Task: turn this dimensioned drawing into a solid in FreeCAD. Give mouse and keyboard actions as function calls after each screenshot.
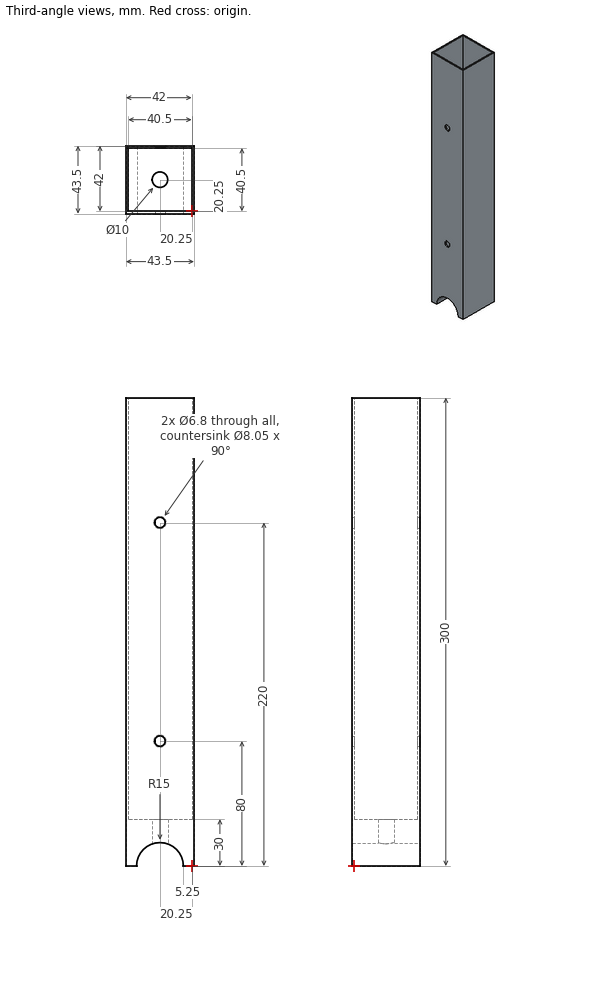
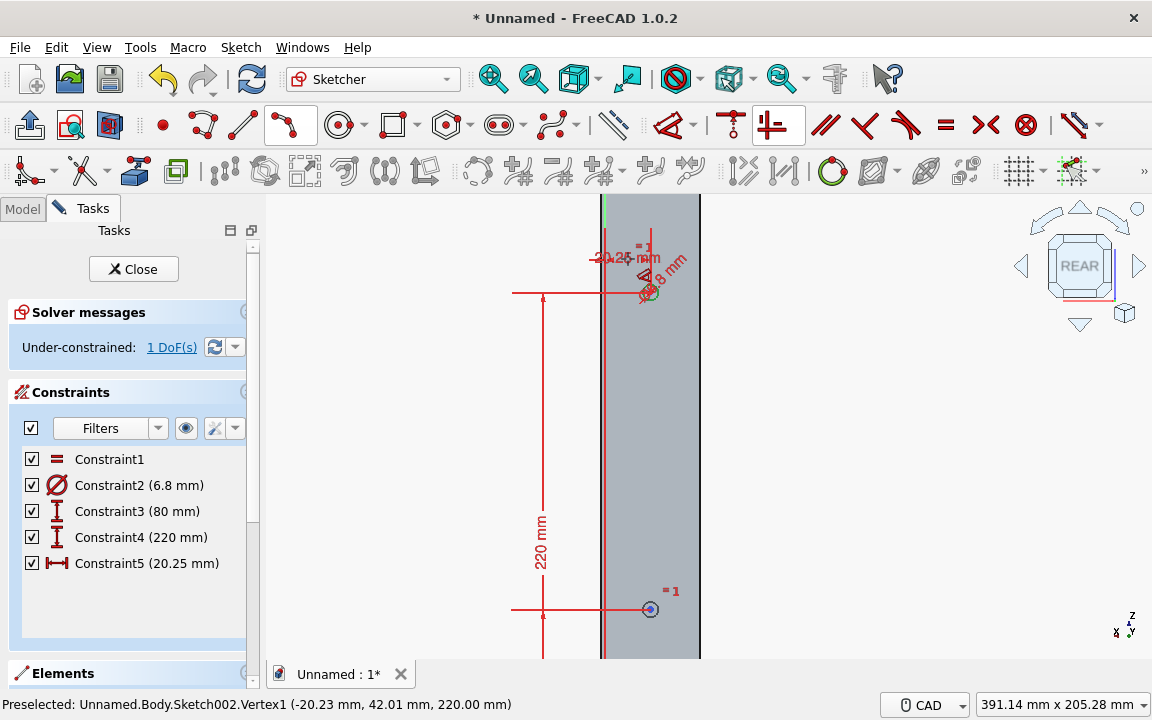
click(651, 610)
click(628, 576)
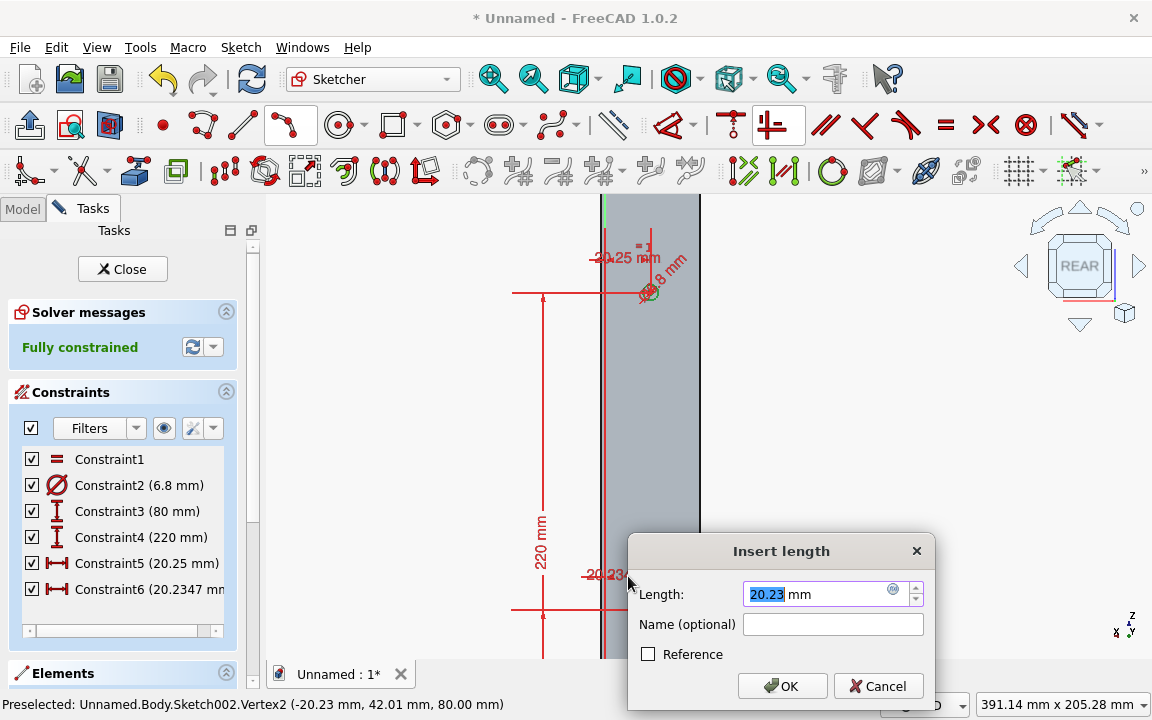
text(20.25)
key(Return)
key(Escape)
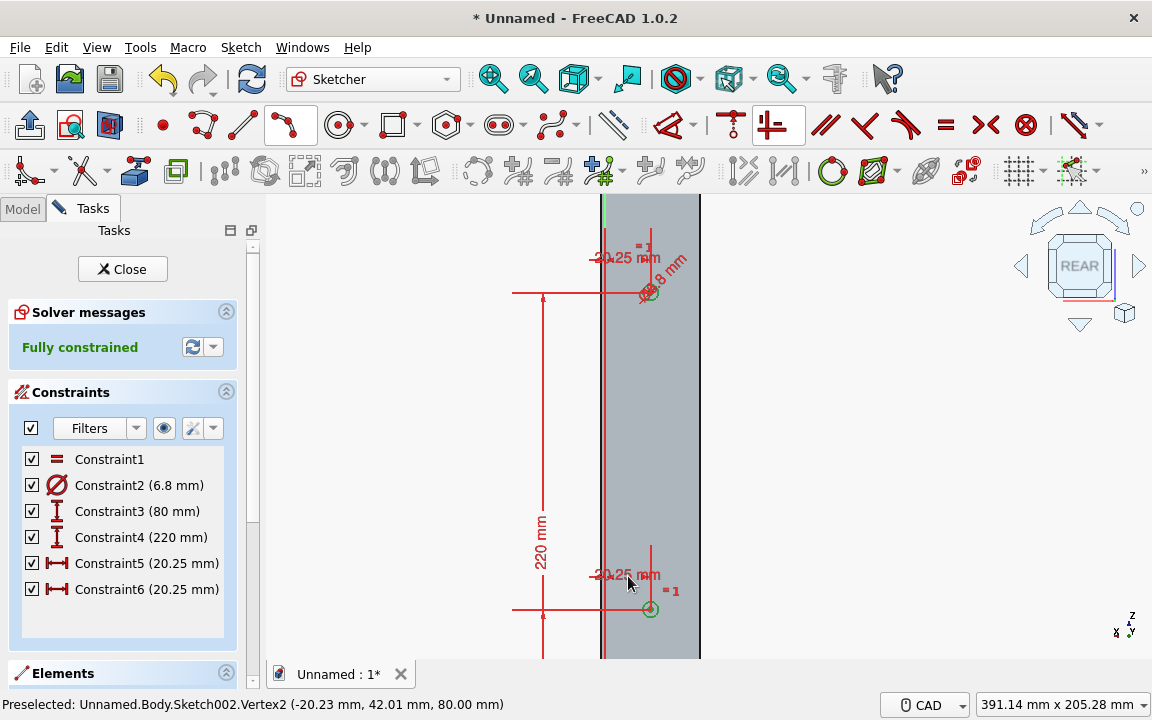
click(123, 269)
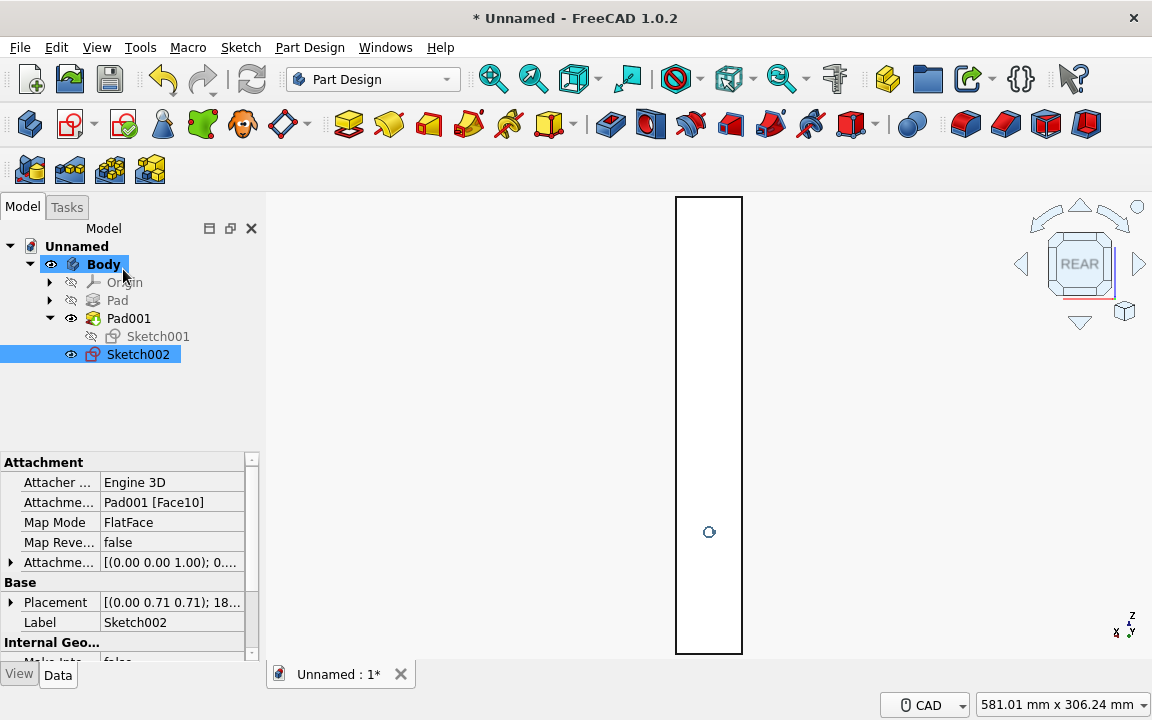
click(652, 124)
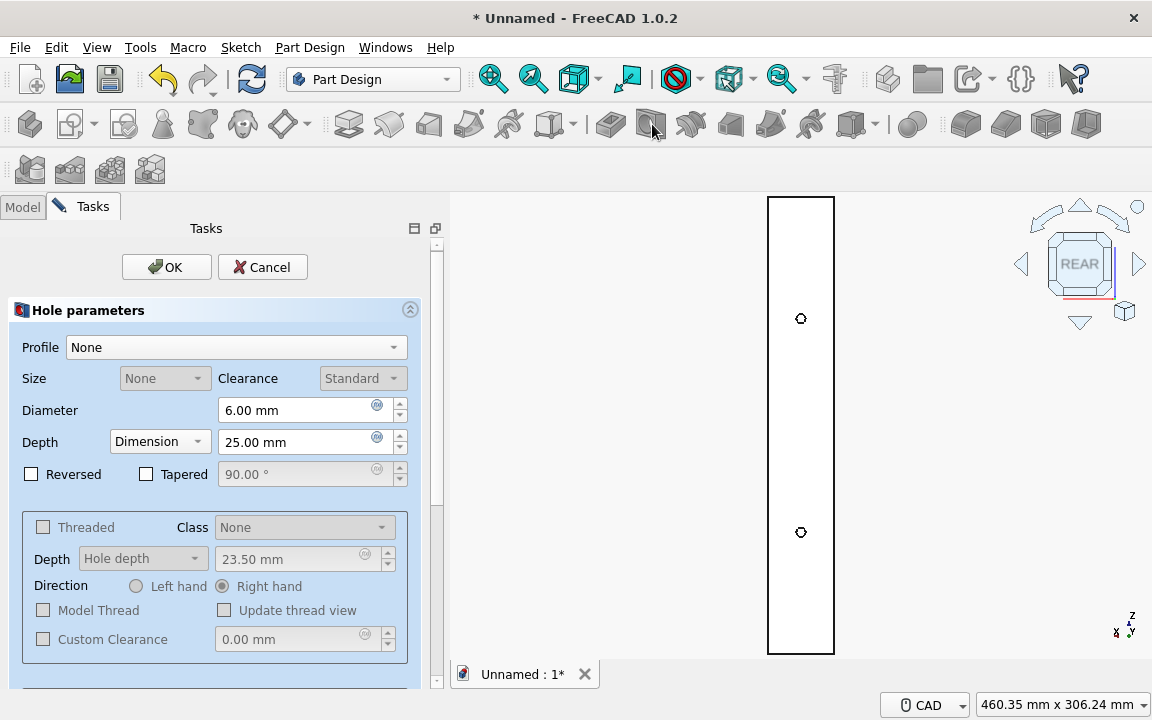
triple_click(305, 410)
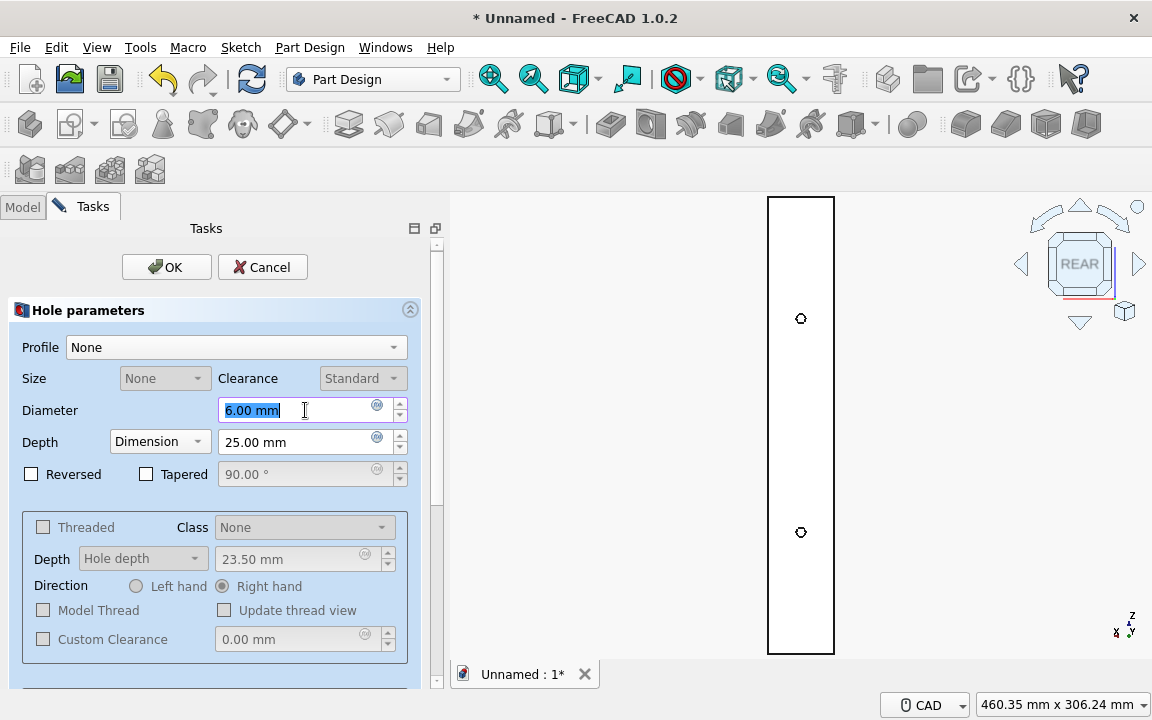
text(6.8)
key(Tab)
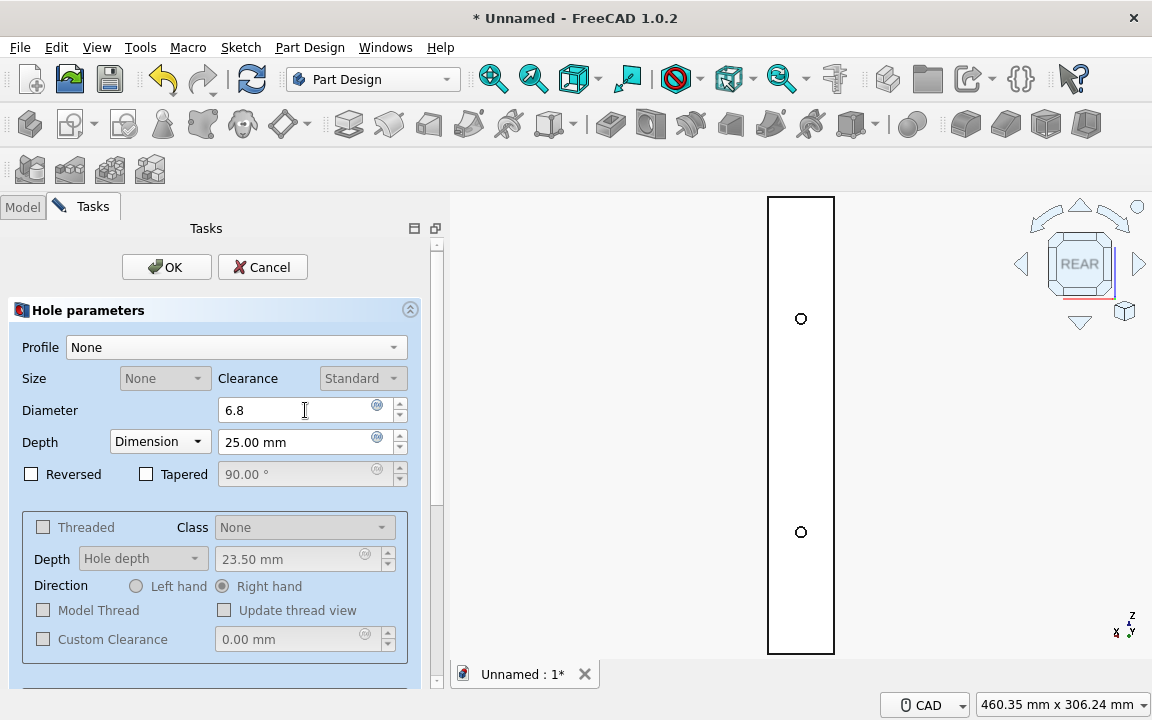
click(161, 442)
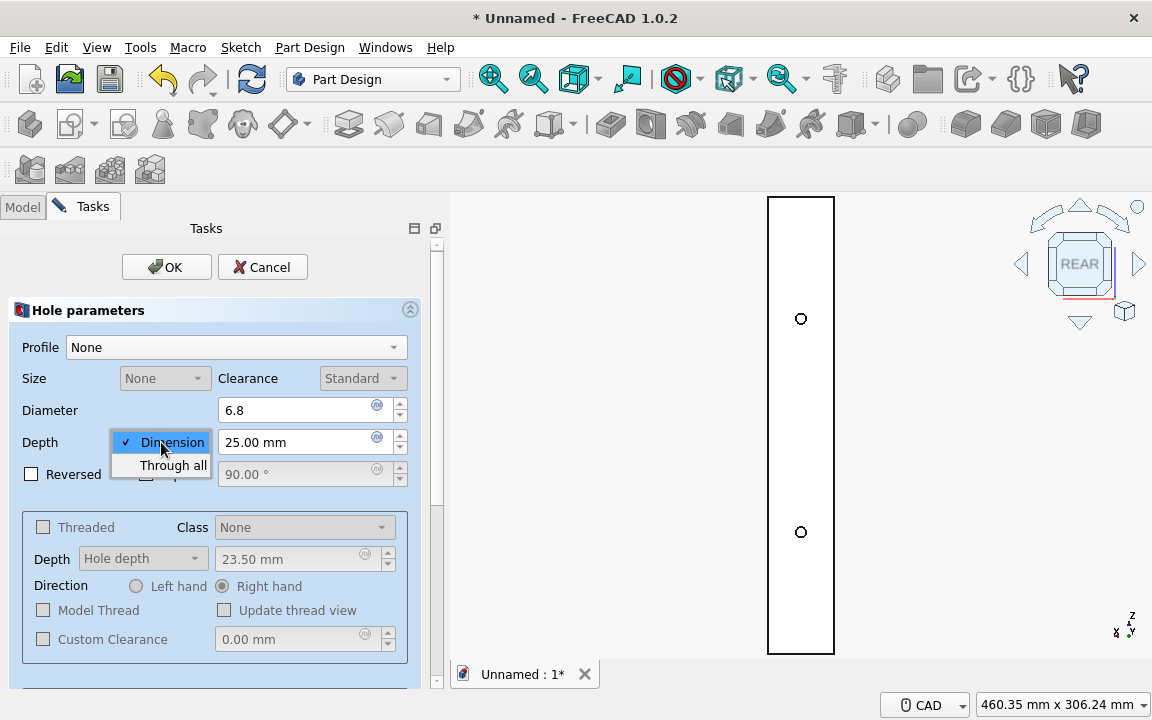
click(160, 466)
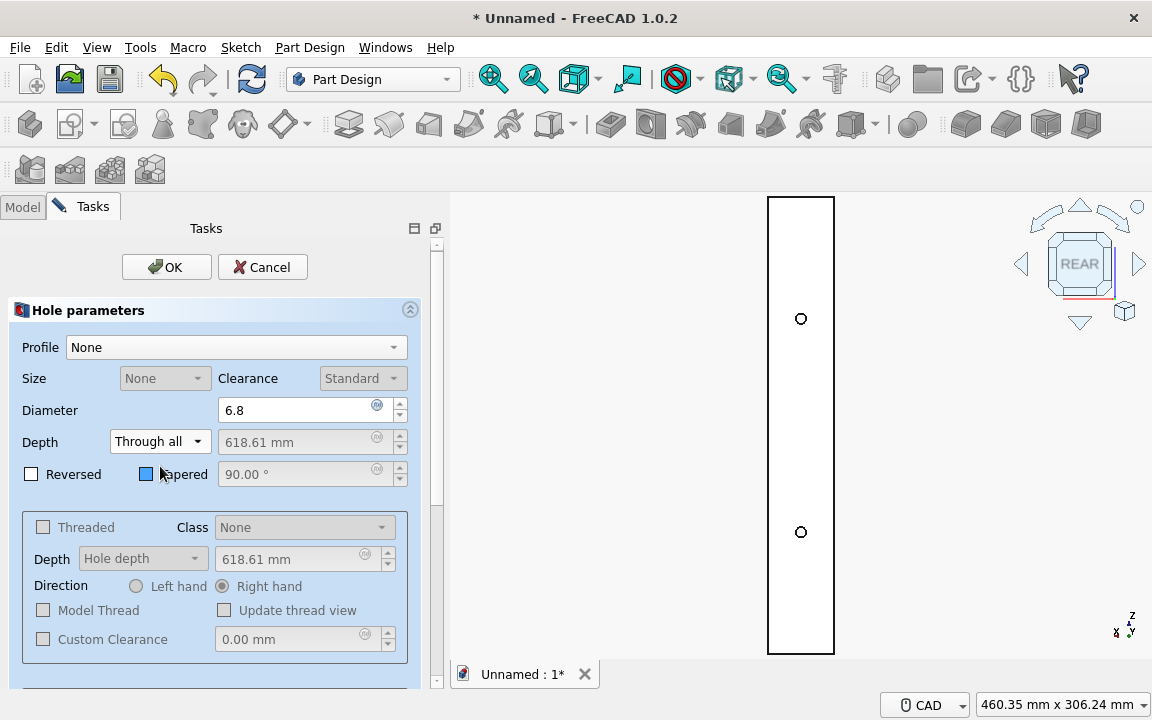
scroll(437, 463, down, 2)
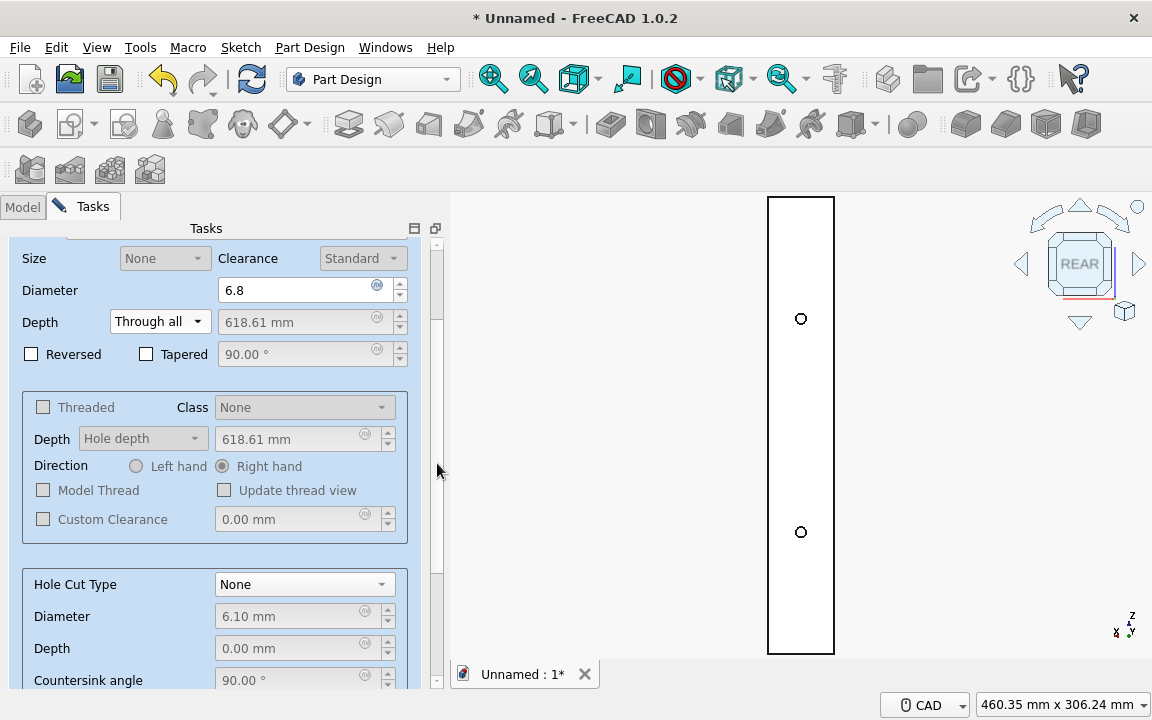
click(306, 584)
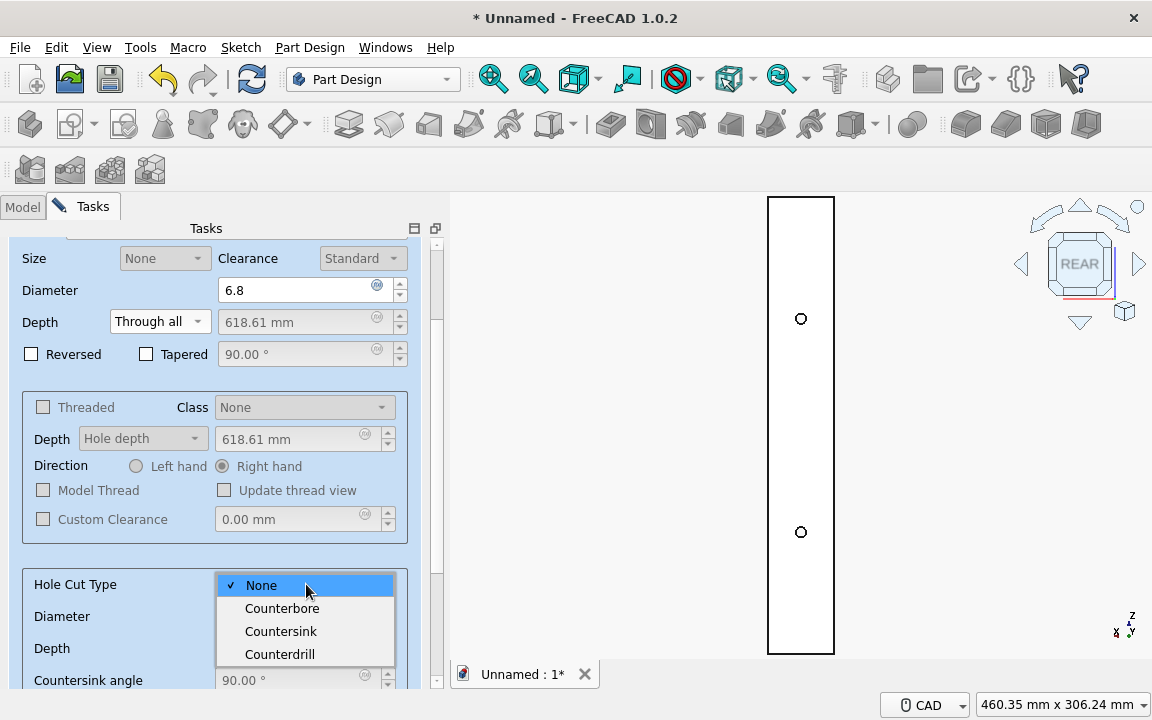
click(304, 632)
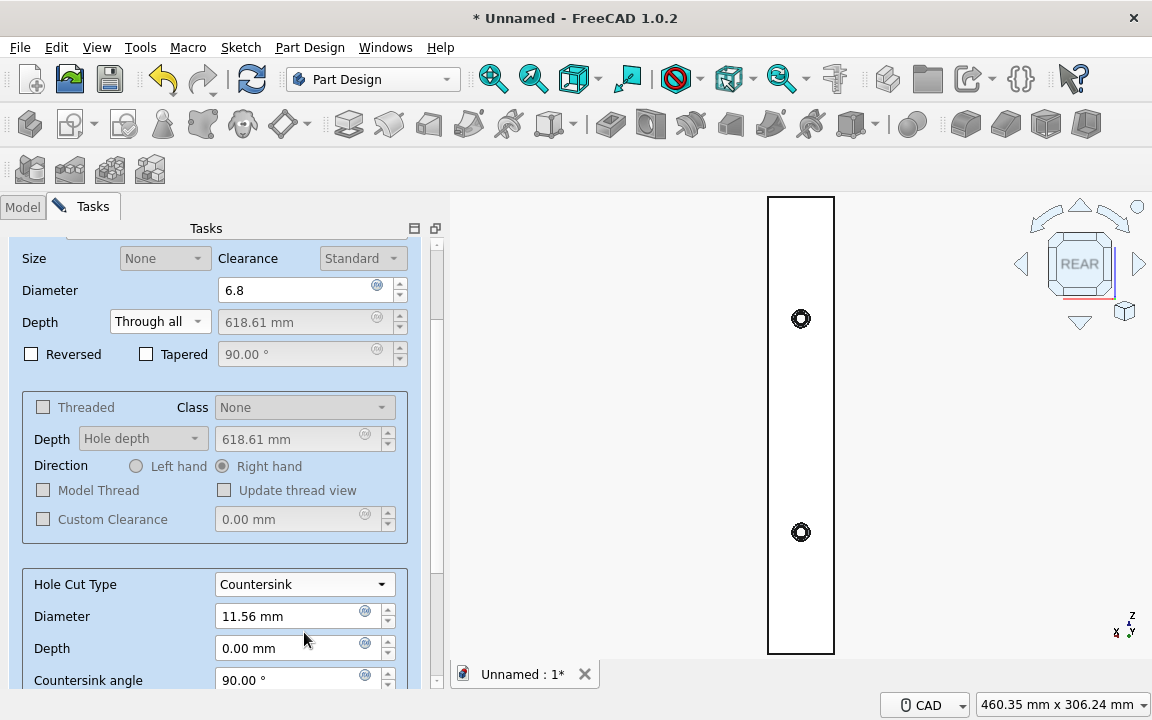
triple_click(298, 616)